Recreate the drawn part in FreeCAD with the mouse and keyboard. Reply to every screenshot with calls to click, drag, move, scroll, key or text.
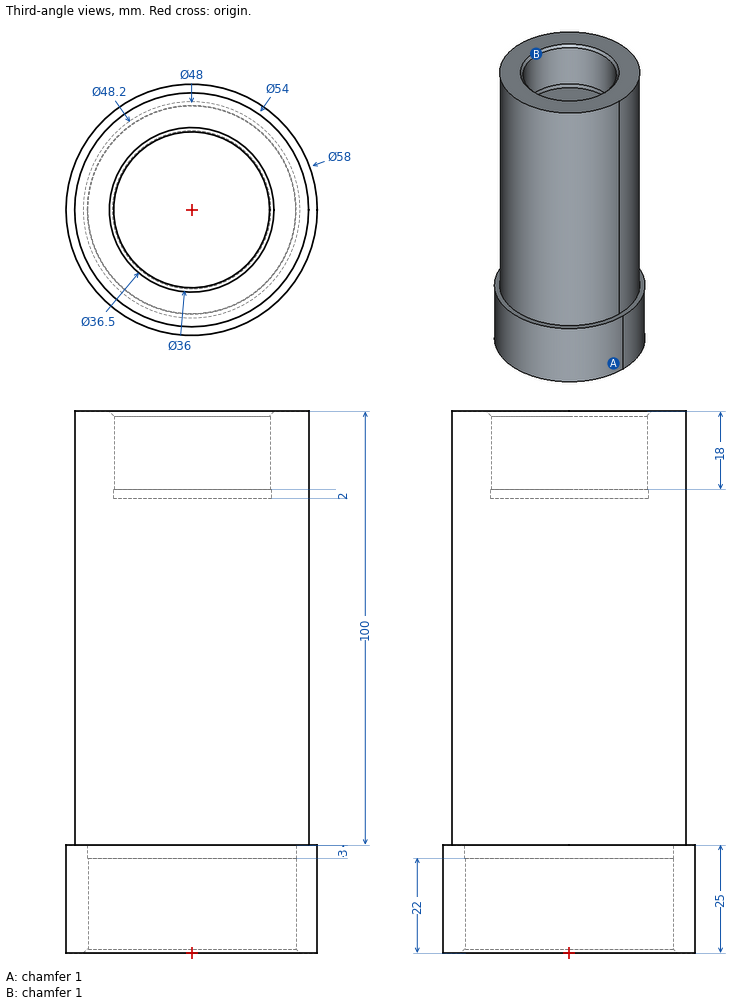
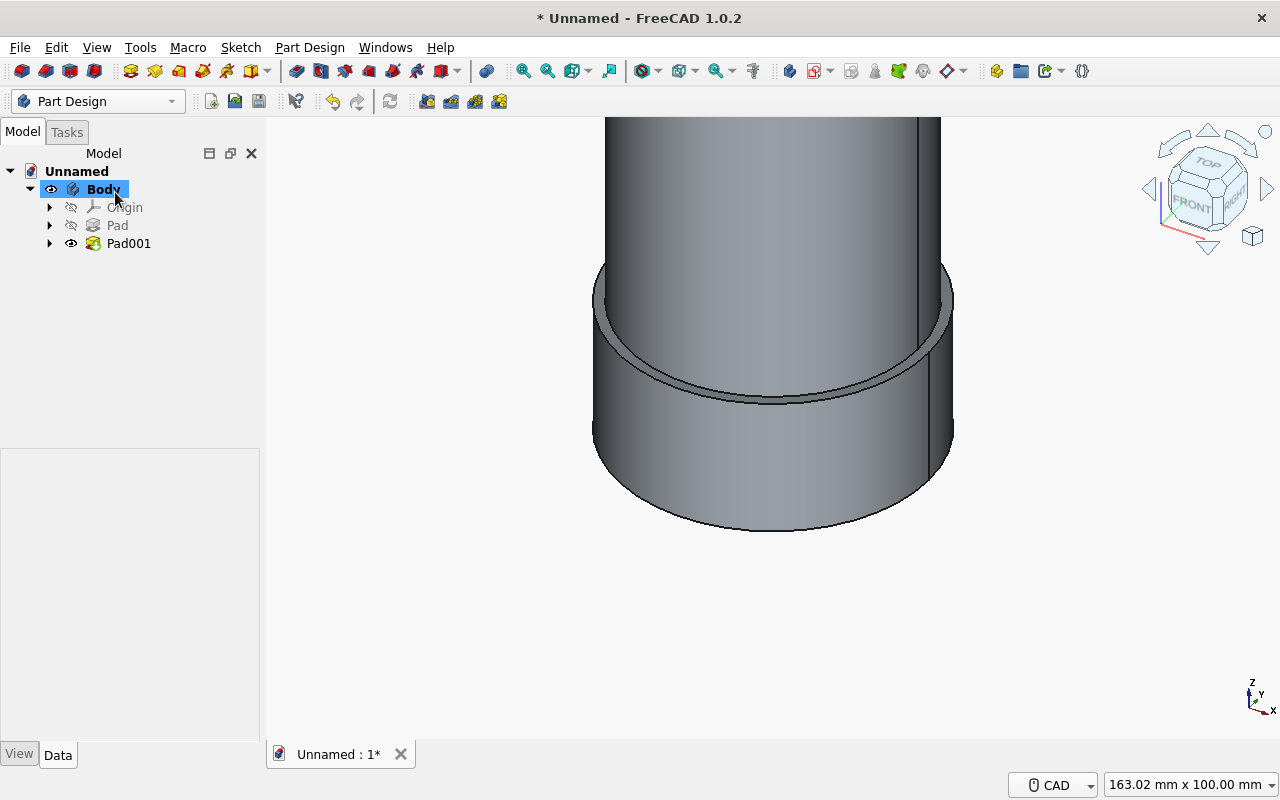
click(524, 72)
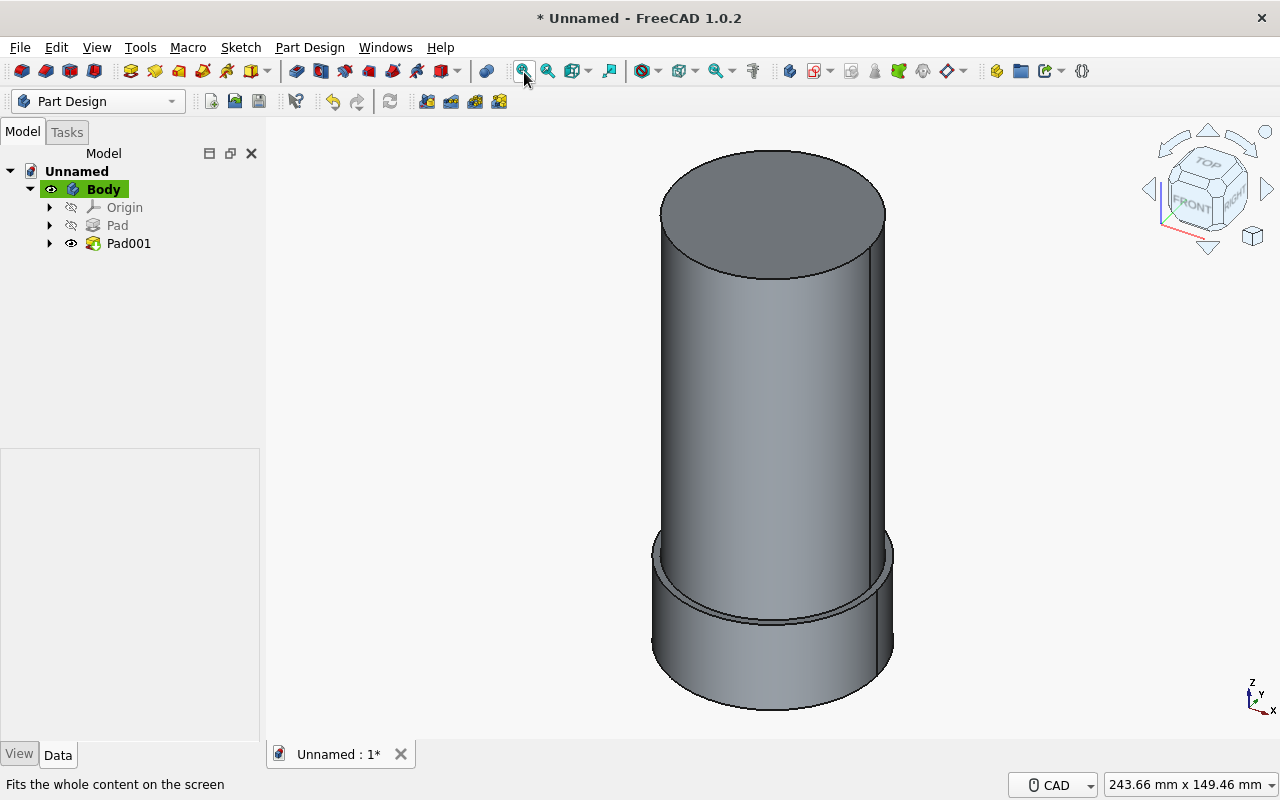
key(5)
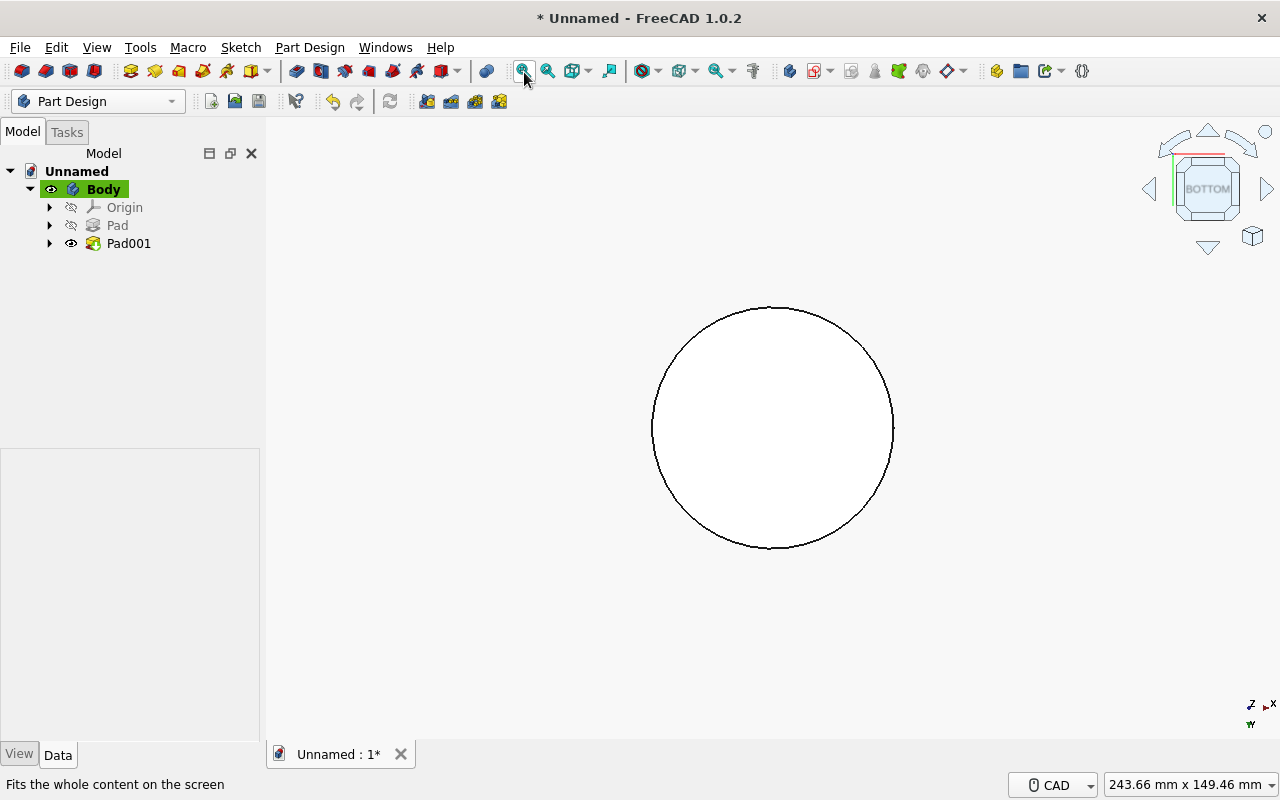
click(524, 72)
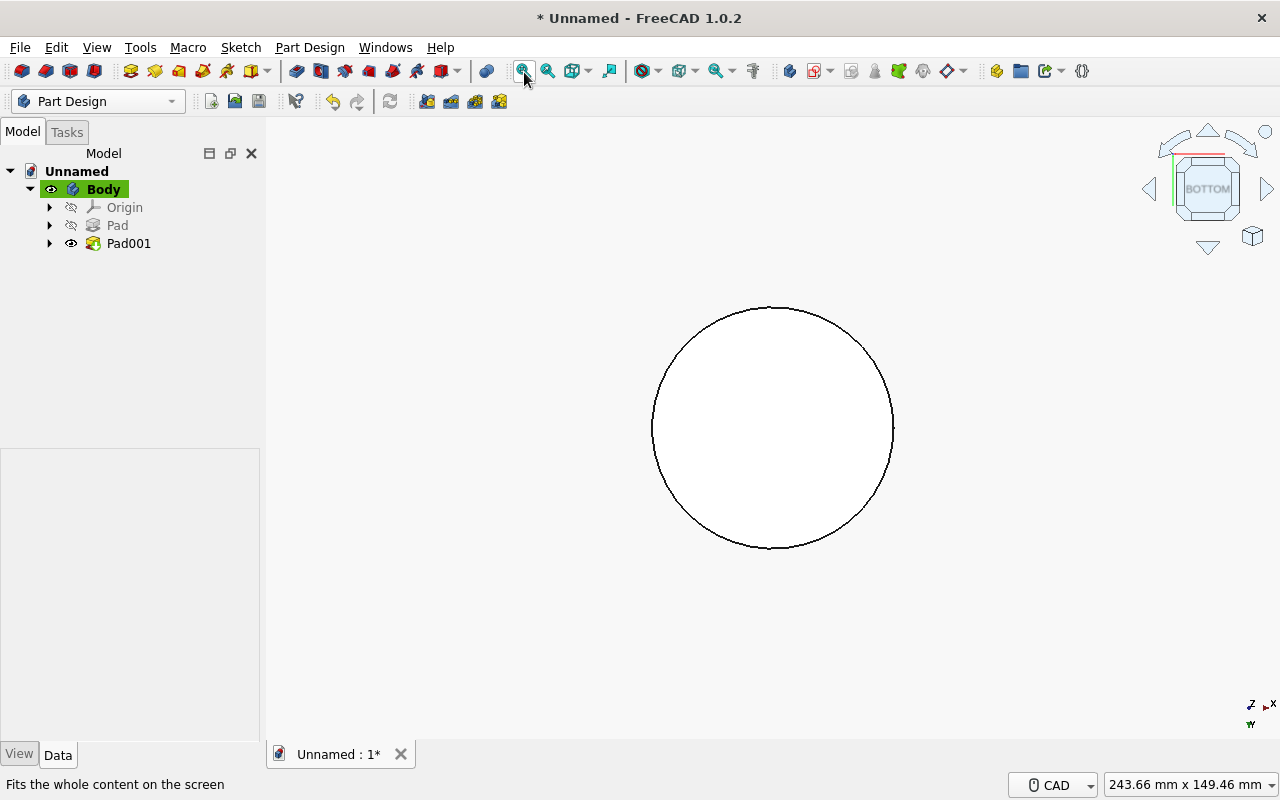
click(773, 427)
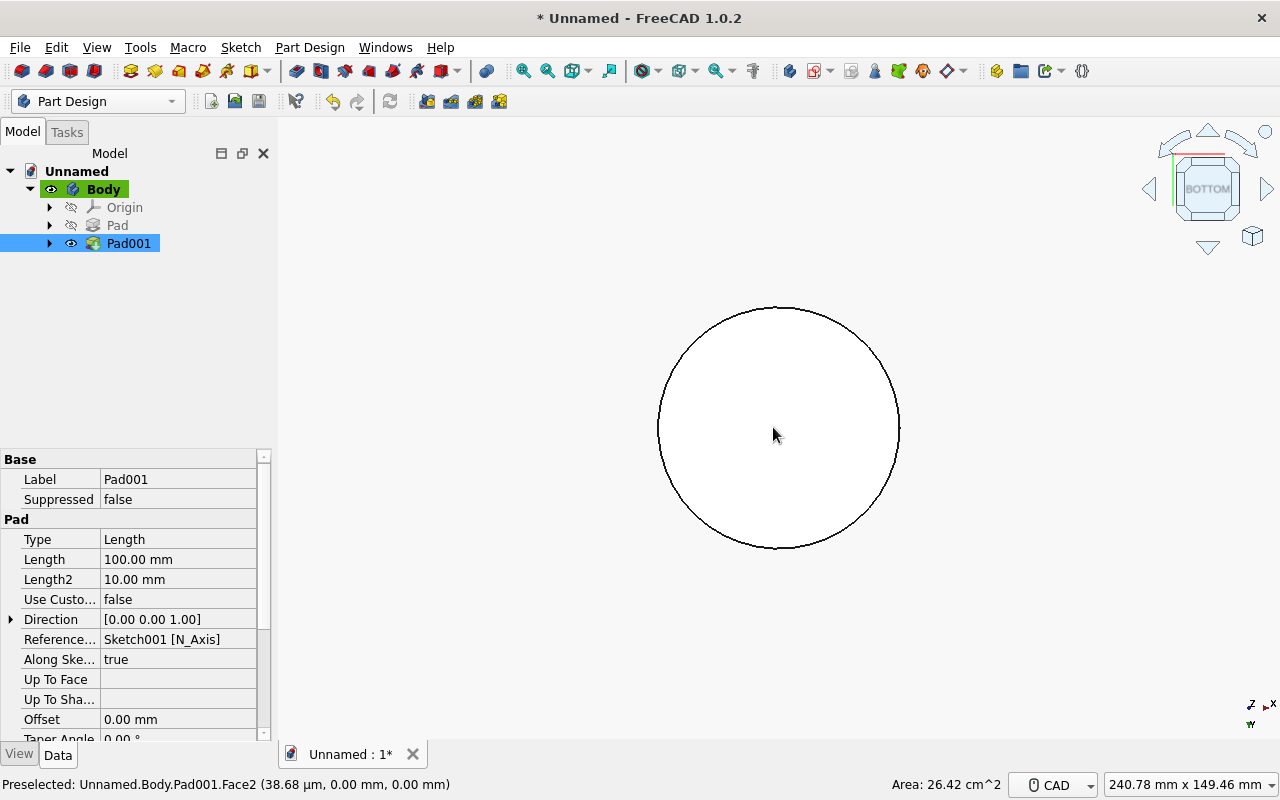
click(814, 72)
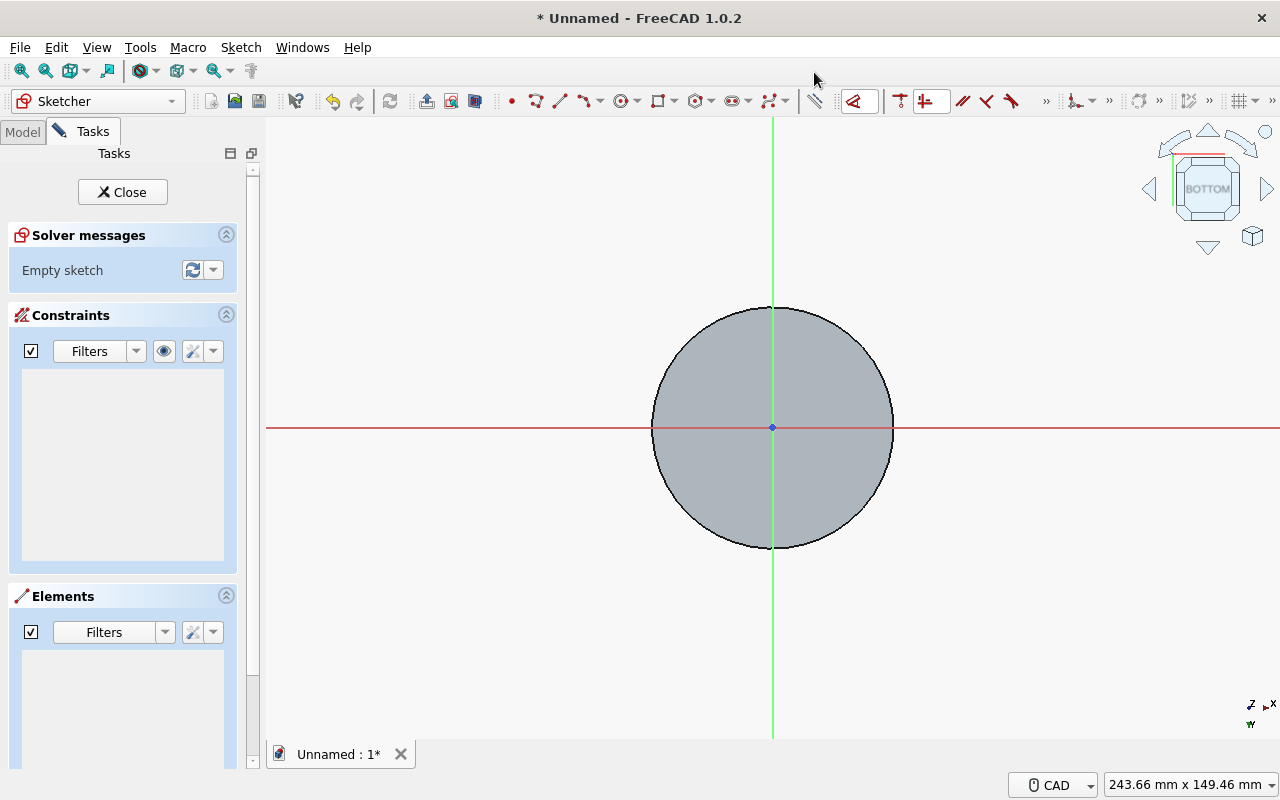
scroll(856, 428, up, 3)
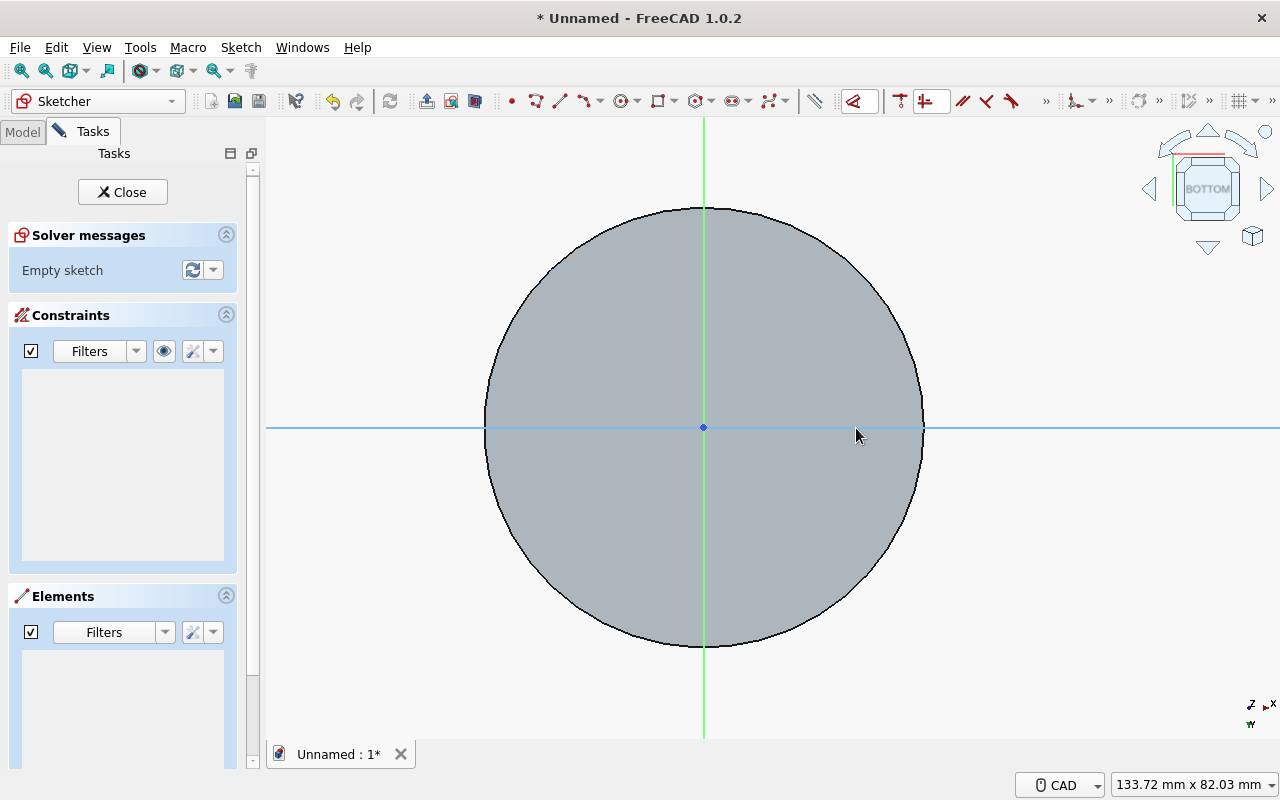
click(622, 102)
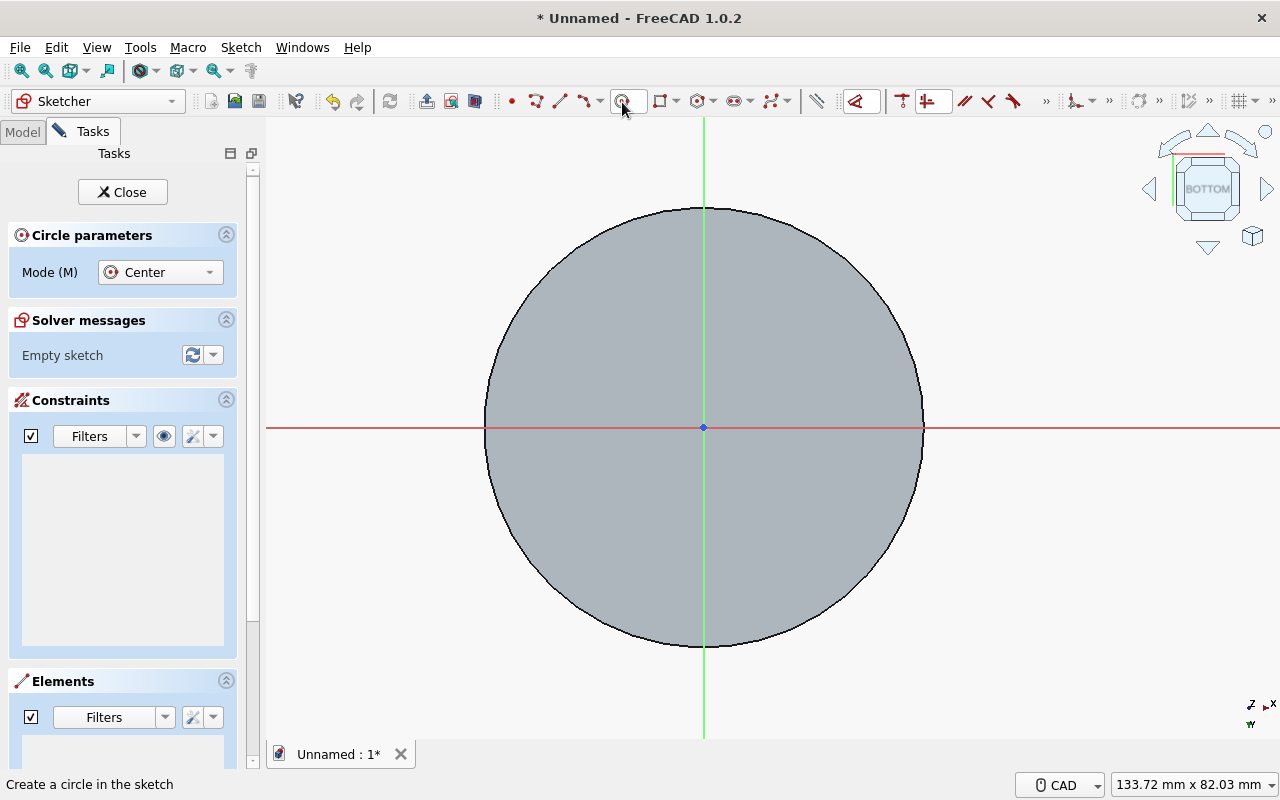
click(704, 428)
move(833, 299)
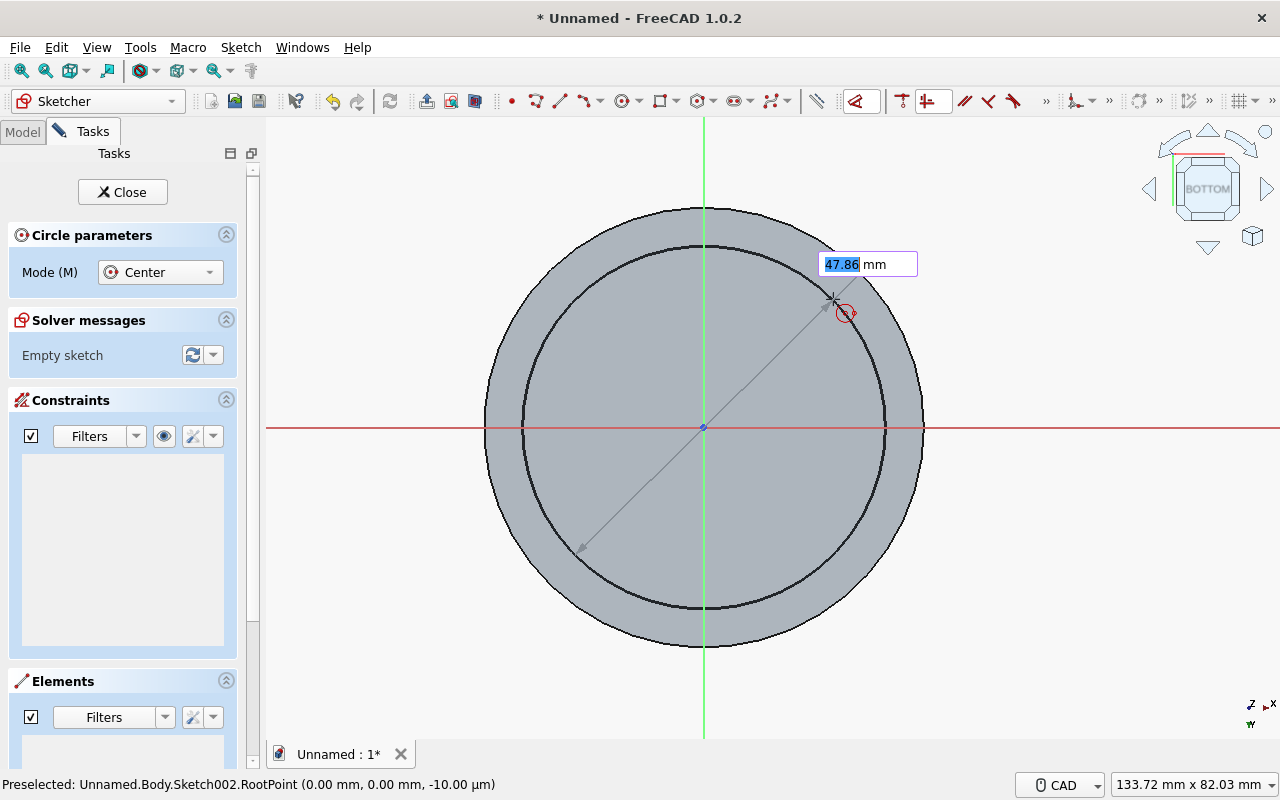
text(48)
key(Return)
key(Escape)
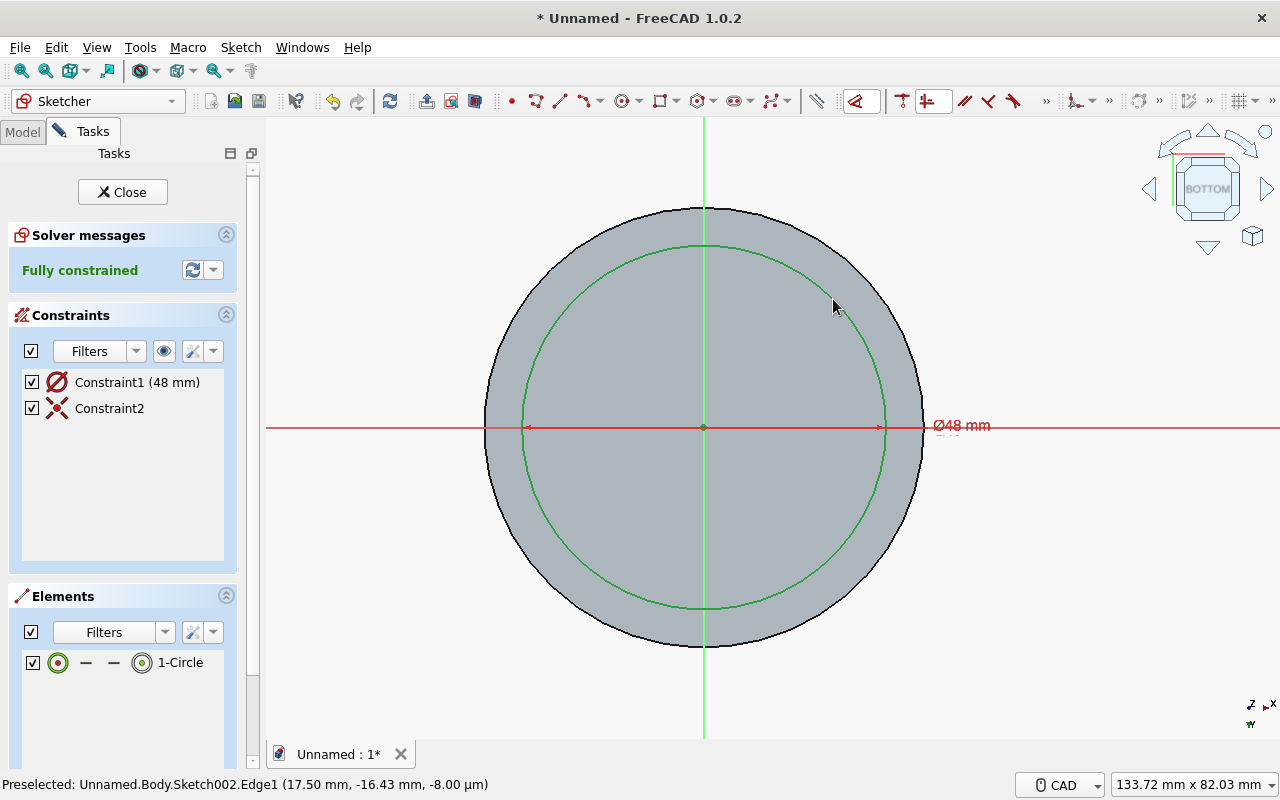
click(123, 192)